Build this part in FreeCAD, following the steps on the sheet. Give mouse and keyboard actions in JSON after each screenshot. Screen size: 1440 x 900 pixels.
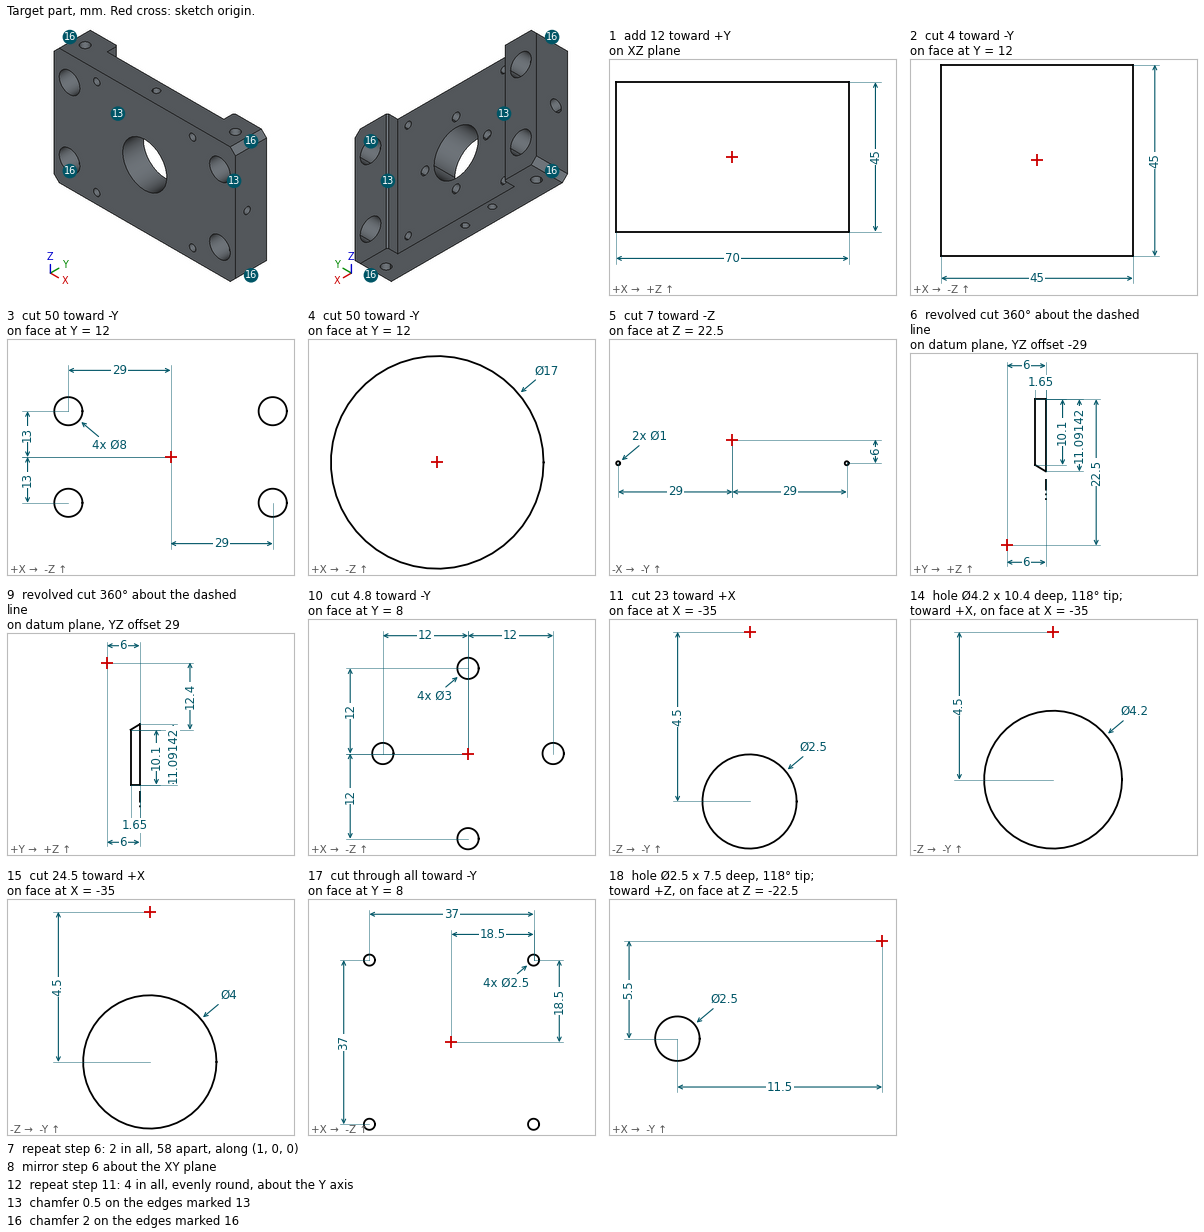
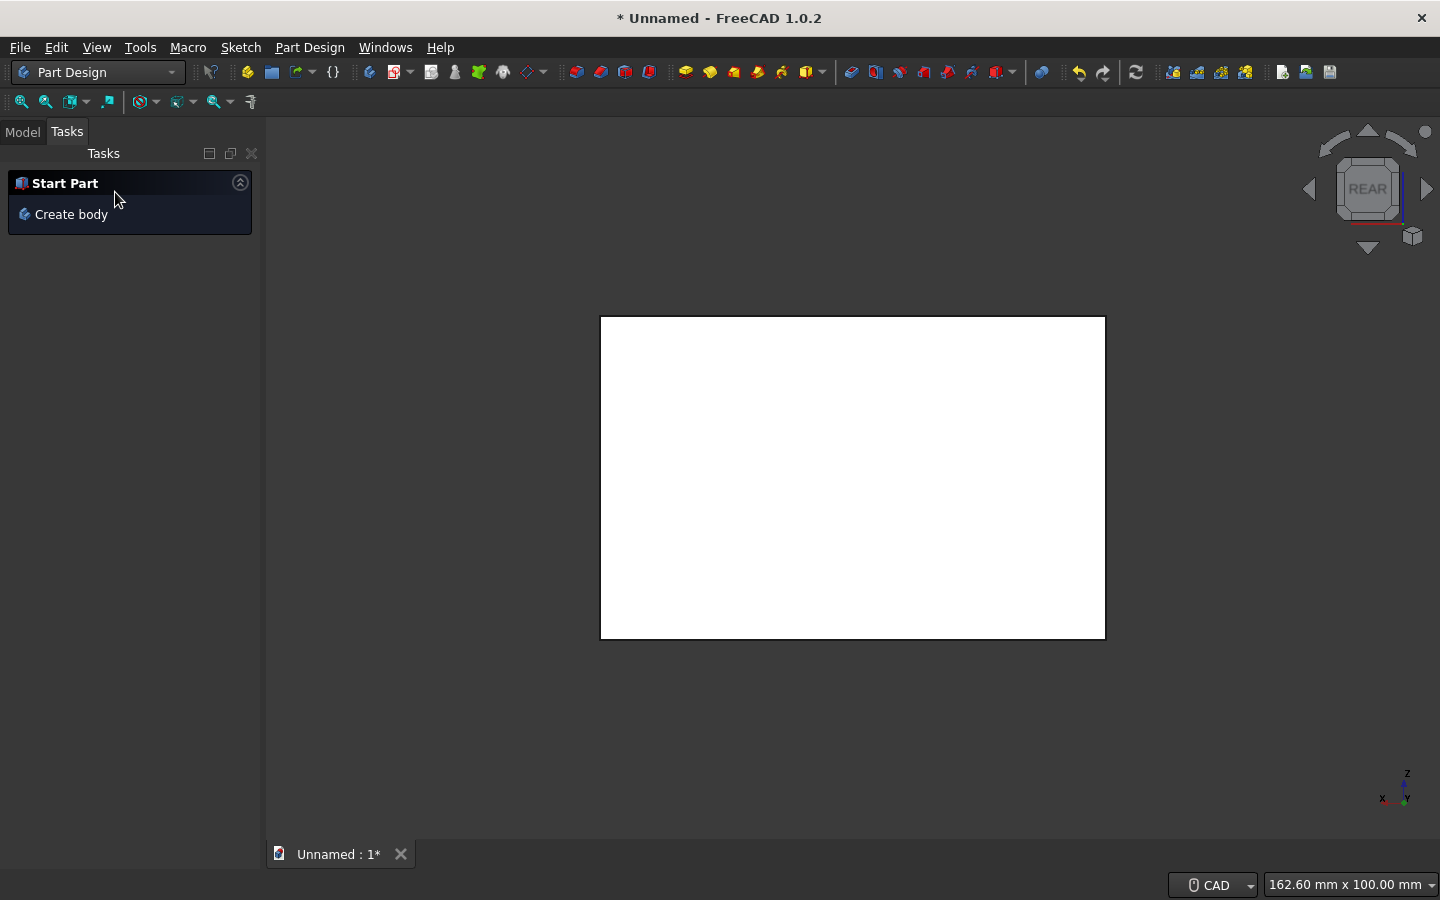
{"action": "left_click", "coordinate": [22, 102]}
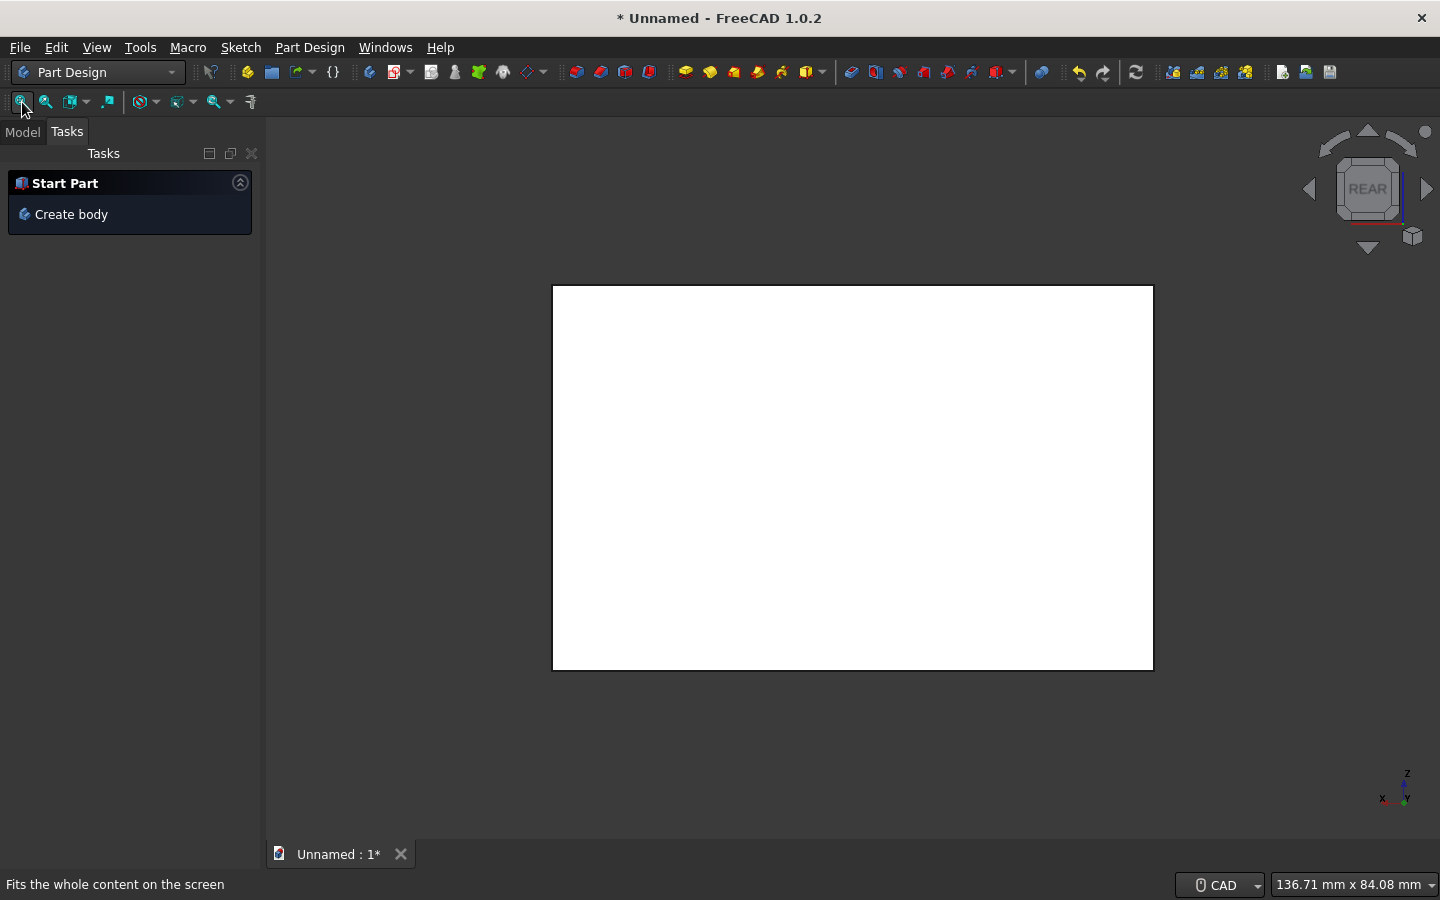
{"action": "left_click", "coordinate": [767, 477]}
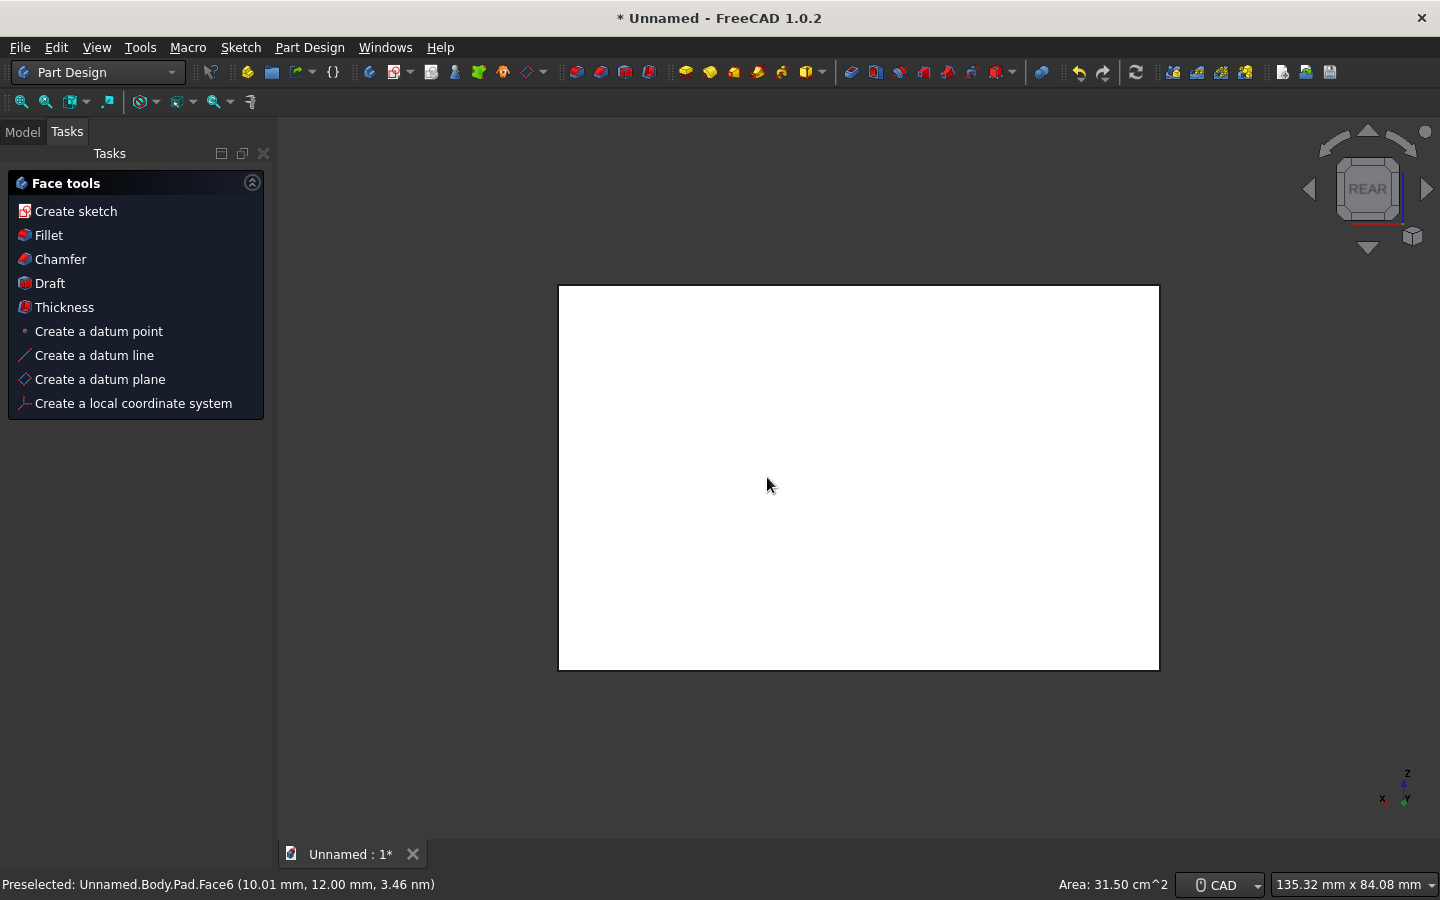
{"action": "left_click", "coordinate": [394, 72]}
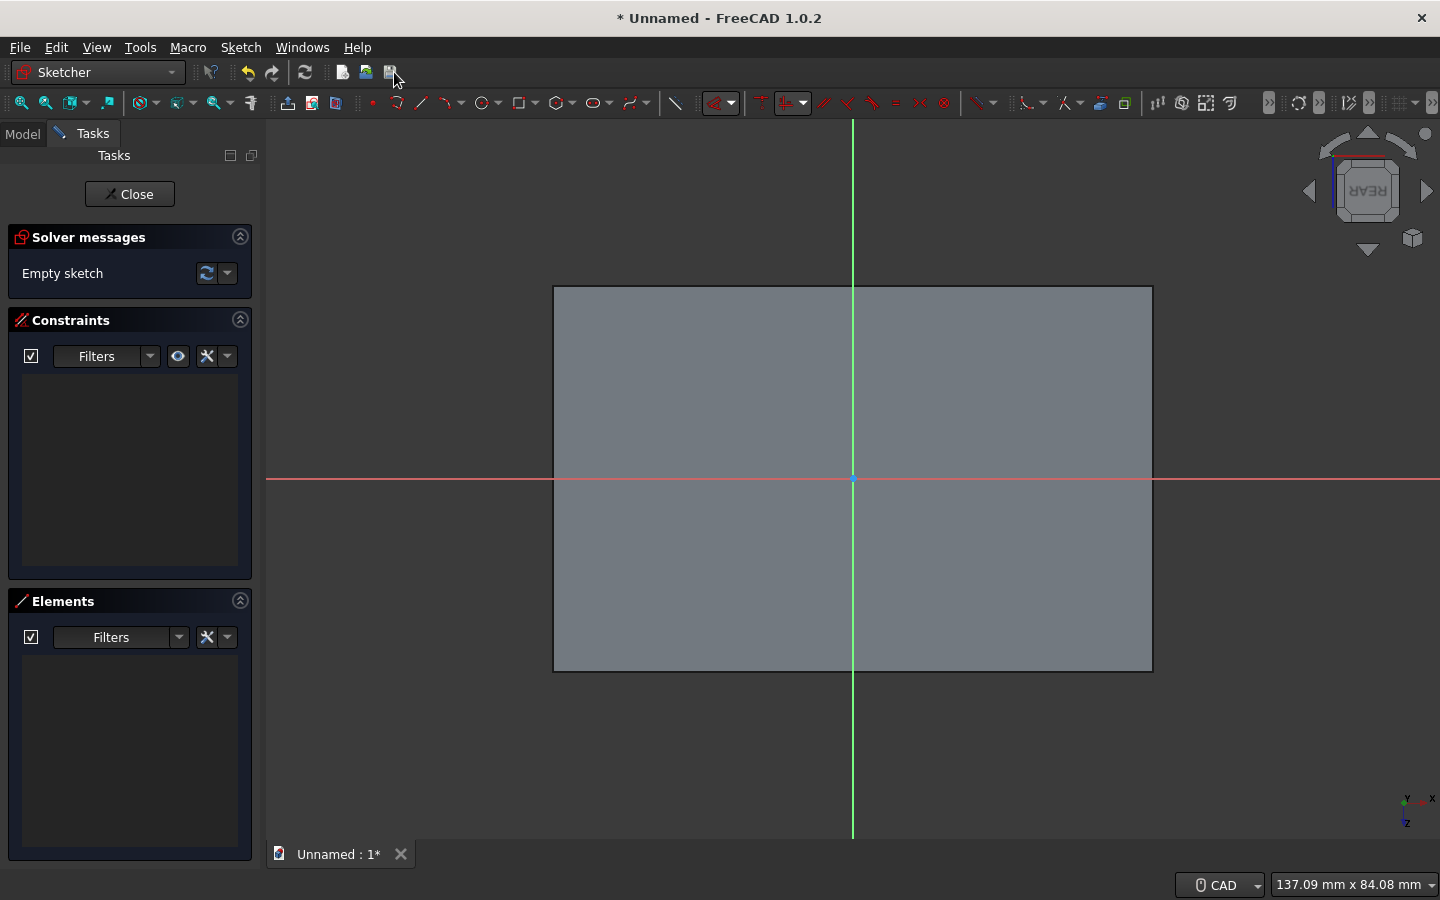
{"action": "left_click", "coordinate": [538, 104]}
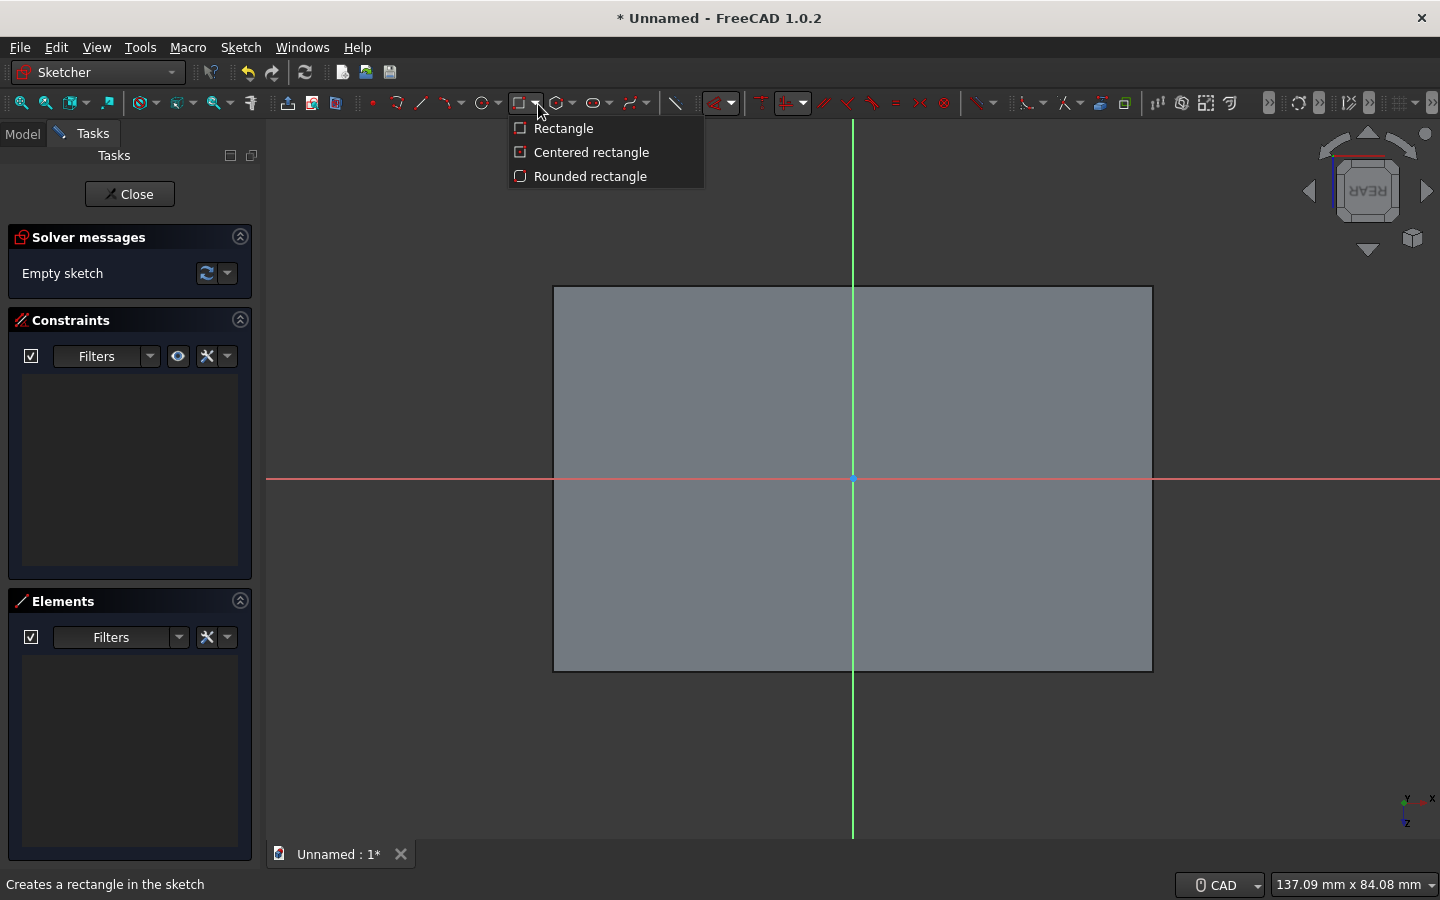
{"action": "left_click", "coordinate": [606, 152]}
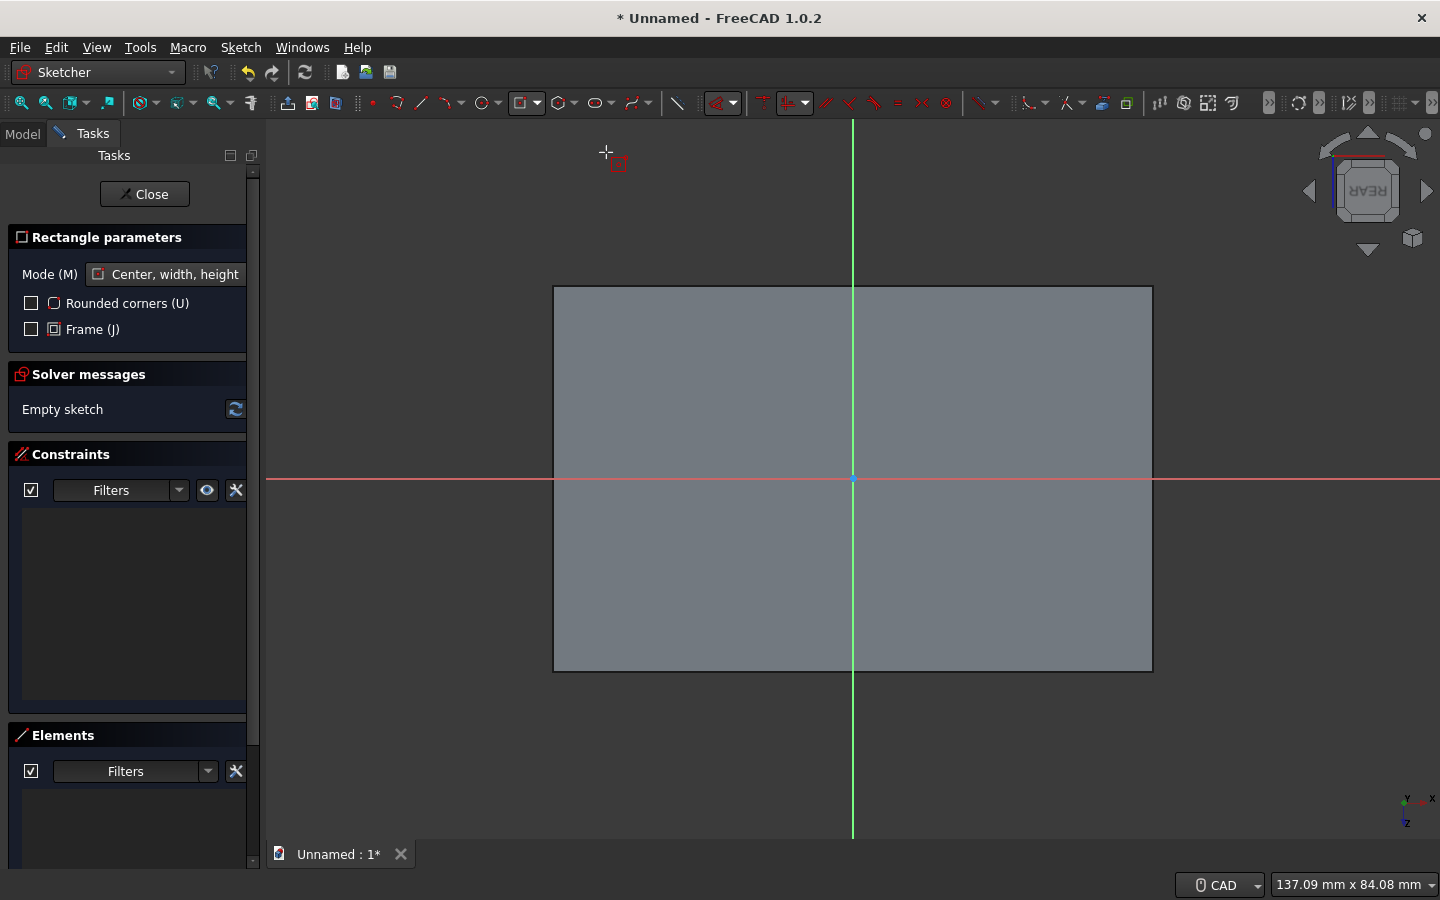
{"action": "left_click", "coordinate": [853, 479]}
{"action": "mouse_move", "coordinate": [1046, 286]}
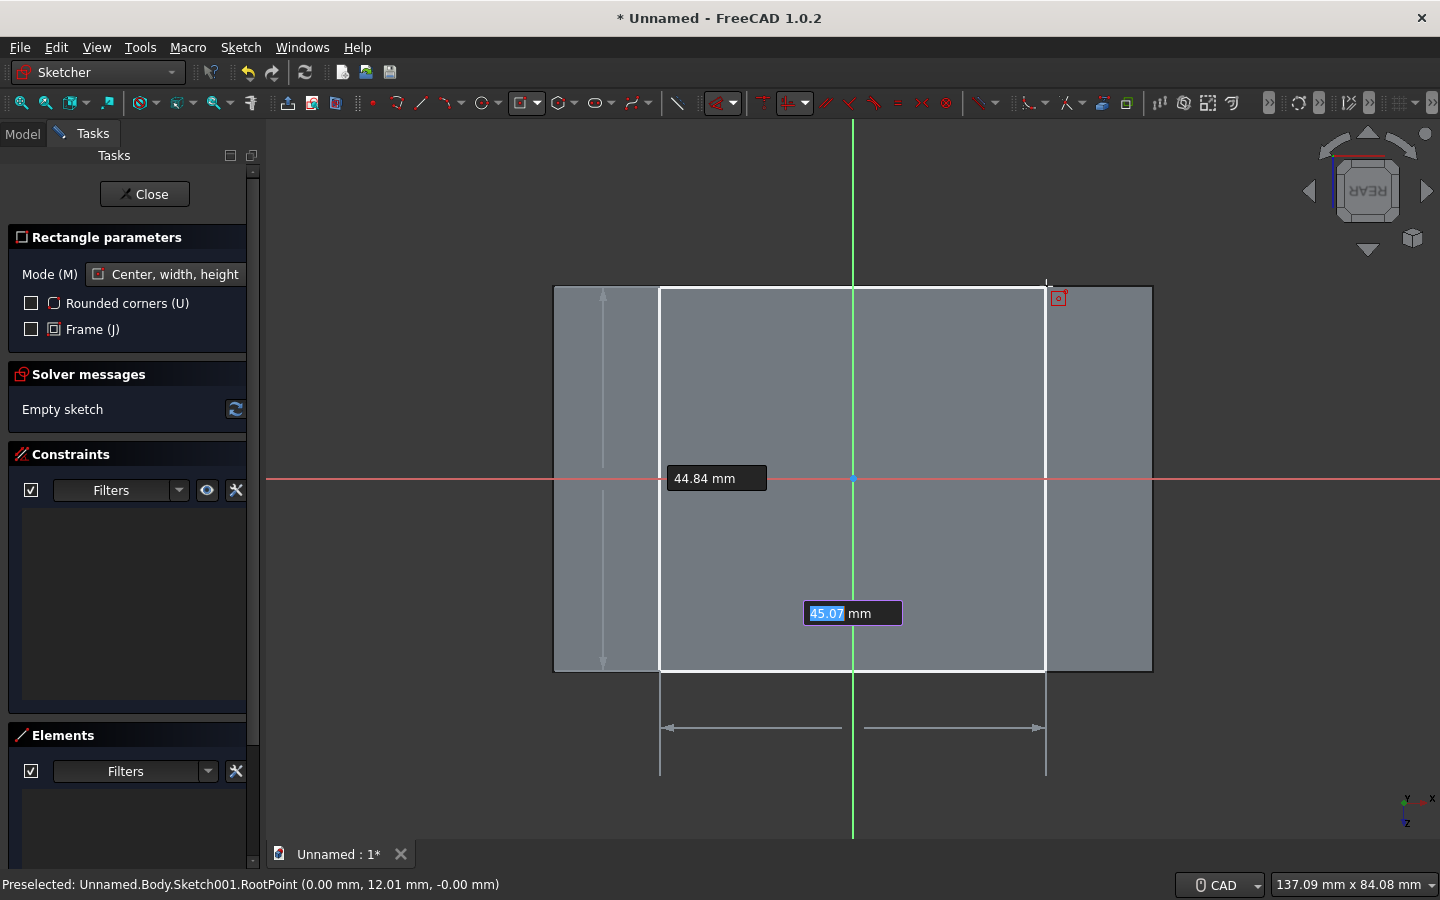
{"action": "type", "text": "45"}
{"action": "key", "text": "Tab"}
{"action": "type", "text": "45"}
{"action": "key", "text": "Return"}
{"action": "key", "text": "Escape"}